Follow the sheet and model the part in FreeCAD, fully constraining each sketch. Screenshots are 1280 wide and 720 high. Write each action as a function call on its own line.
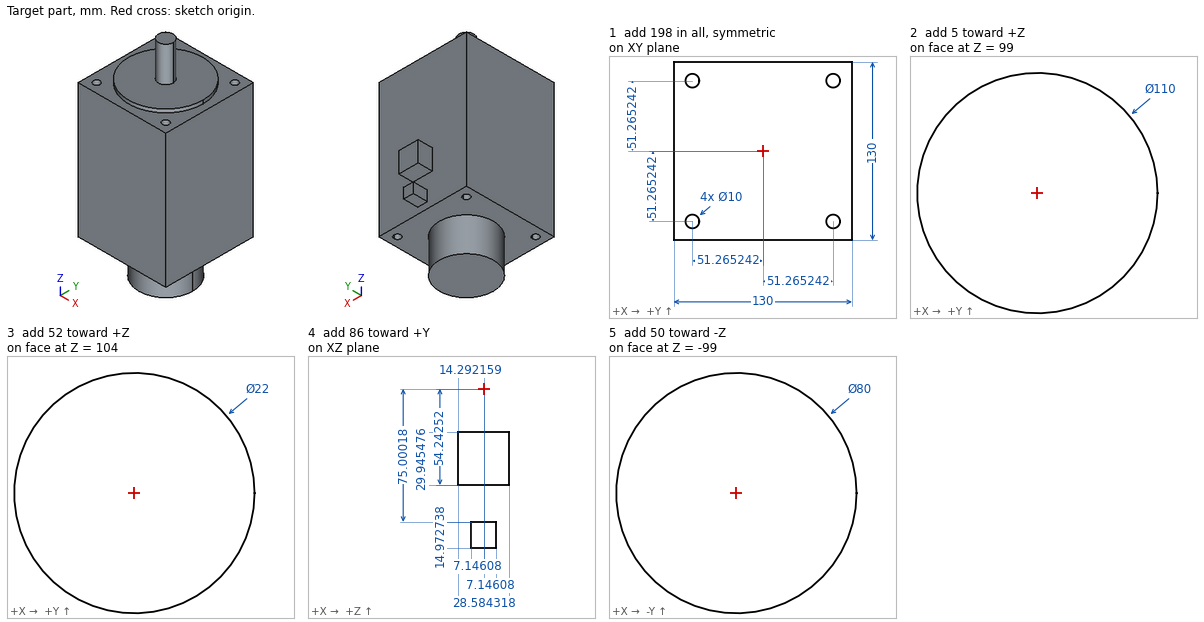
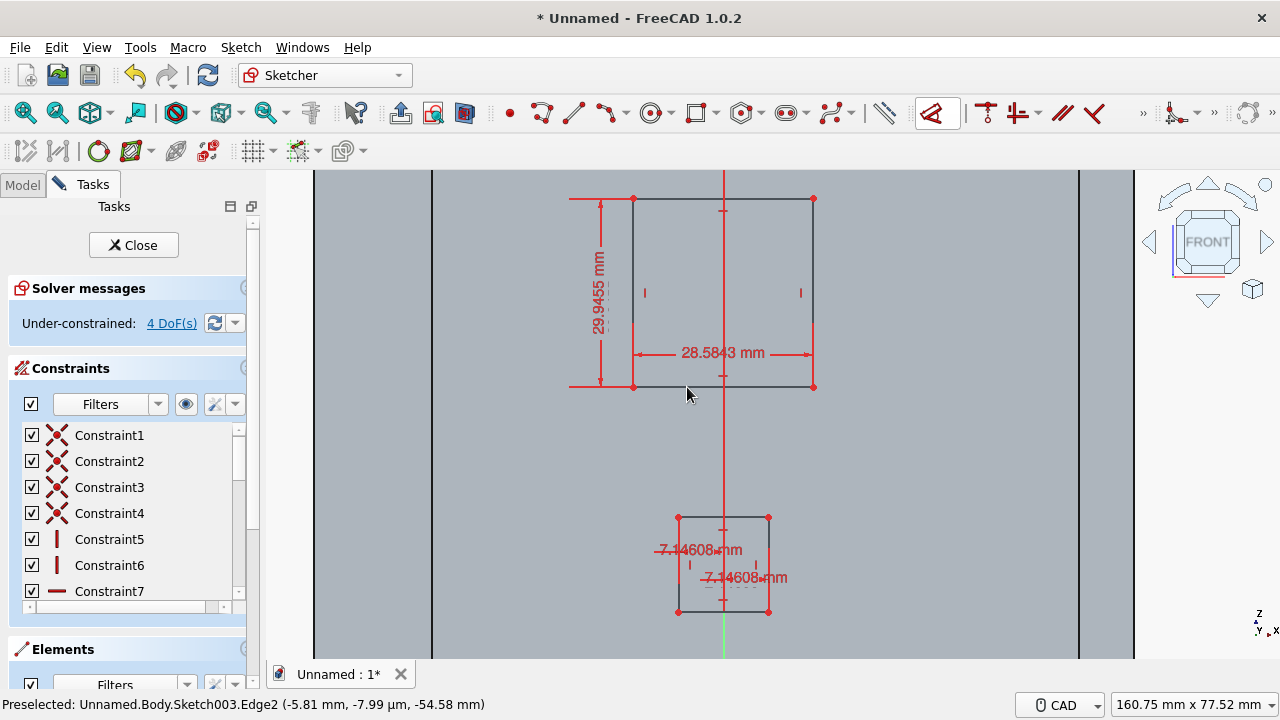
click(679, 584)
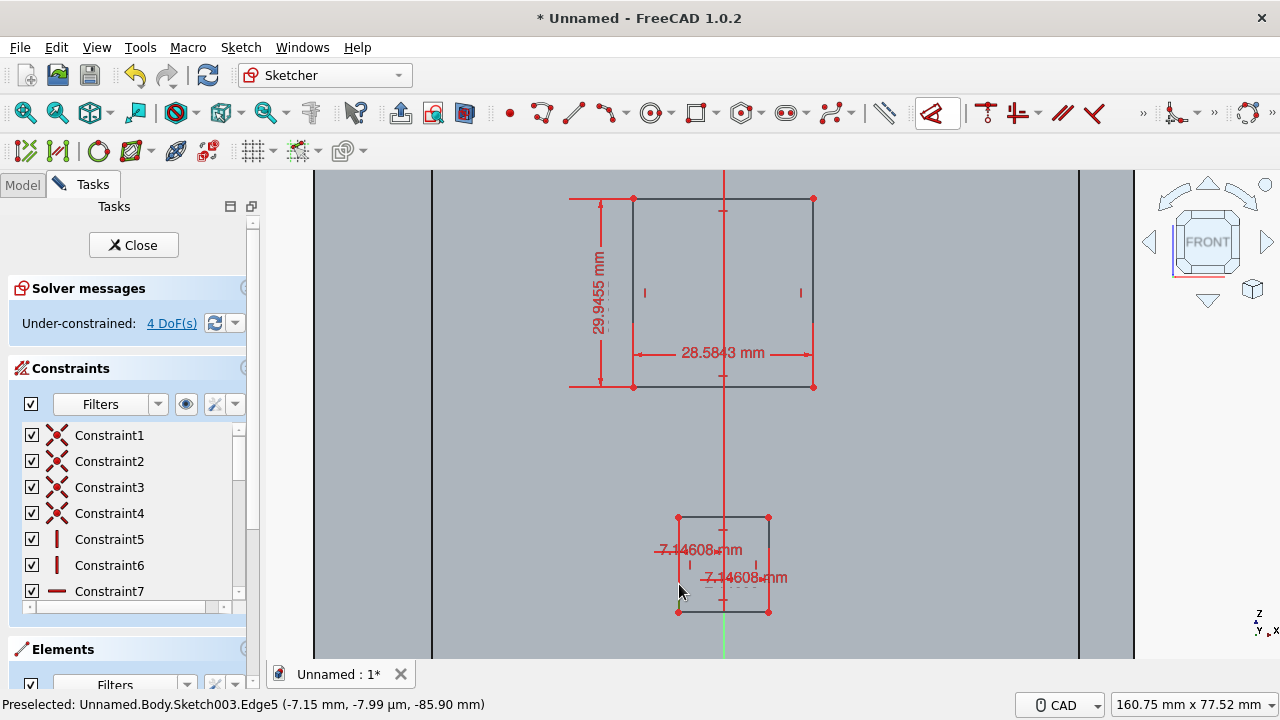
key(i)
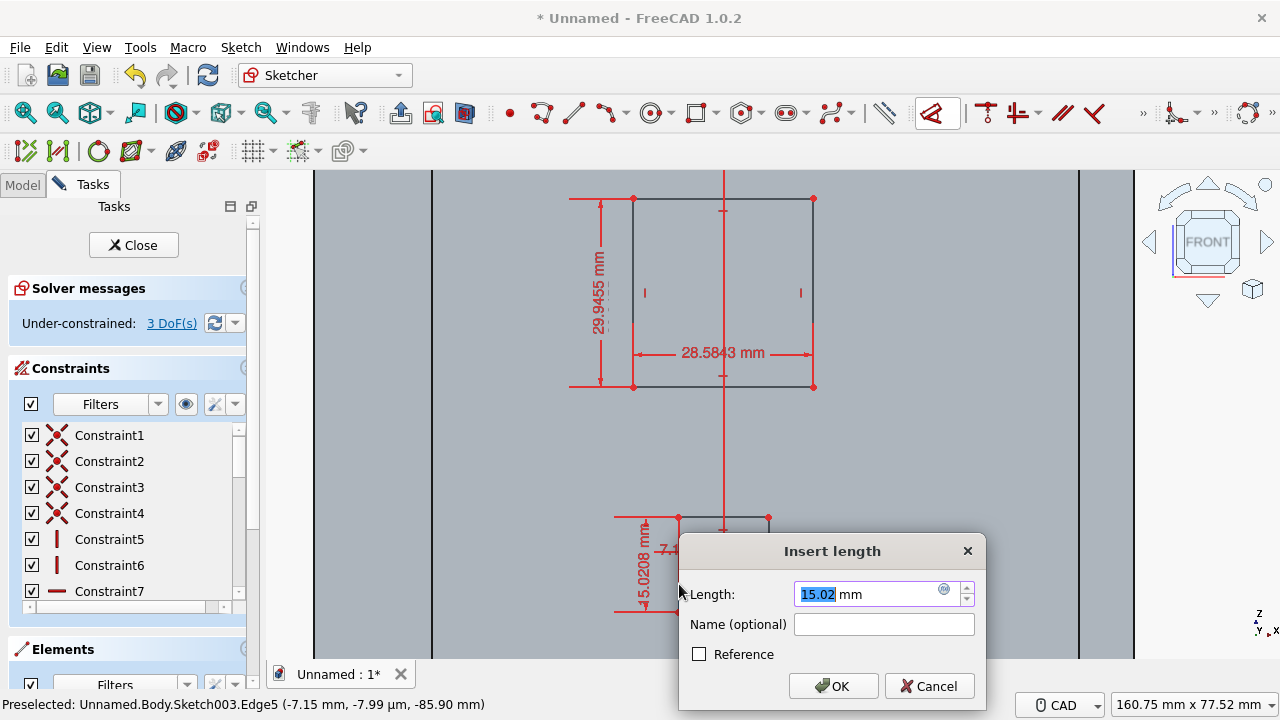
text(14.972738)
key(Return)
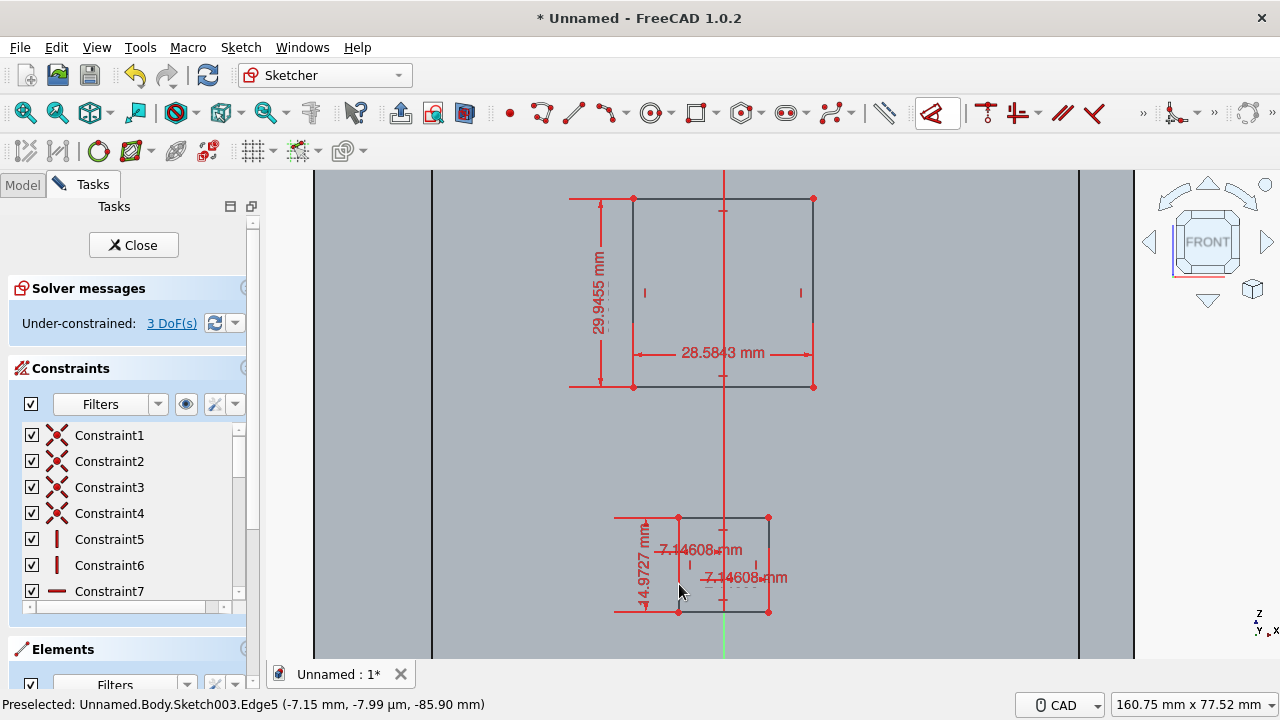
click(633, 387)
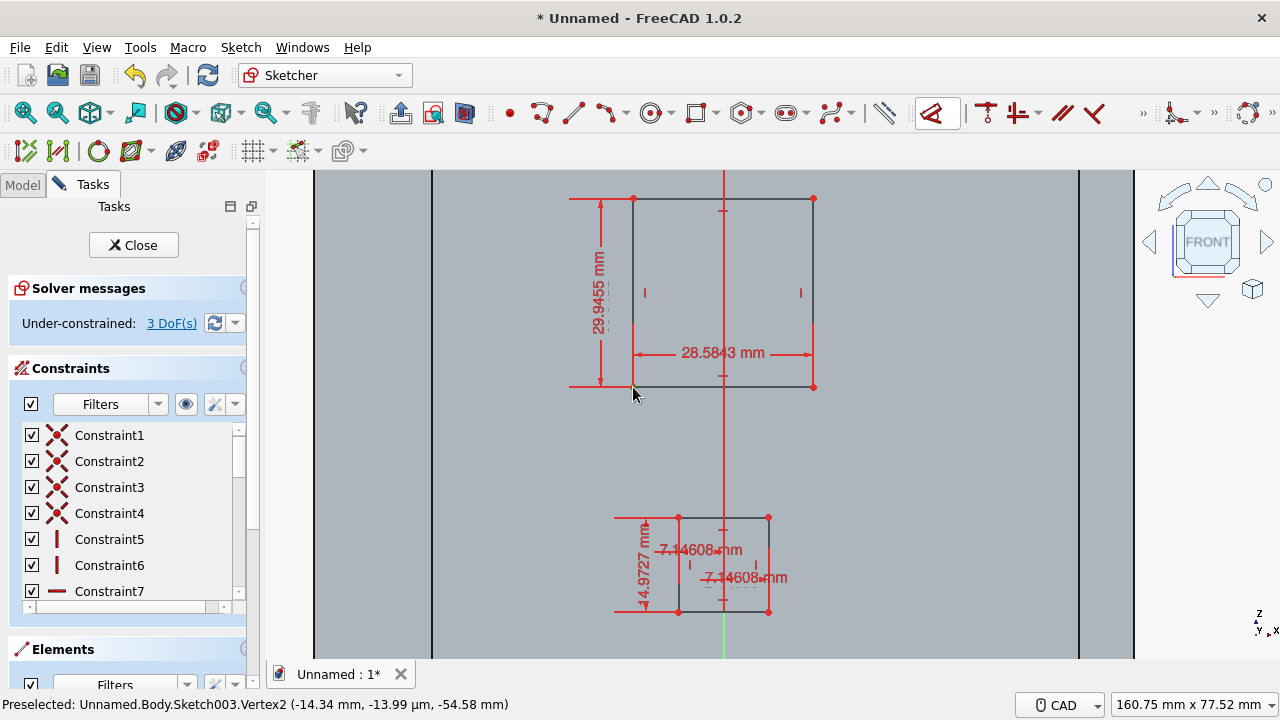
key(i)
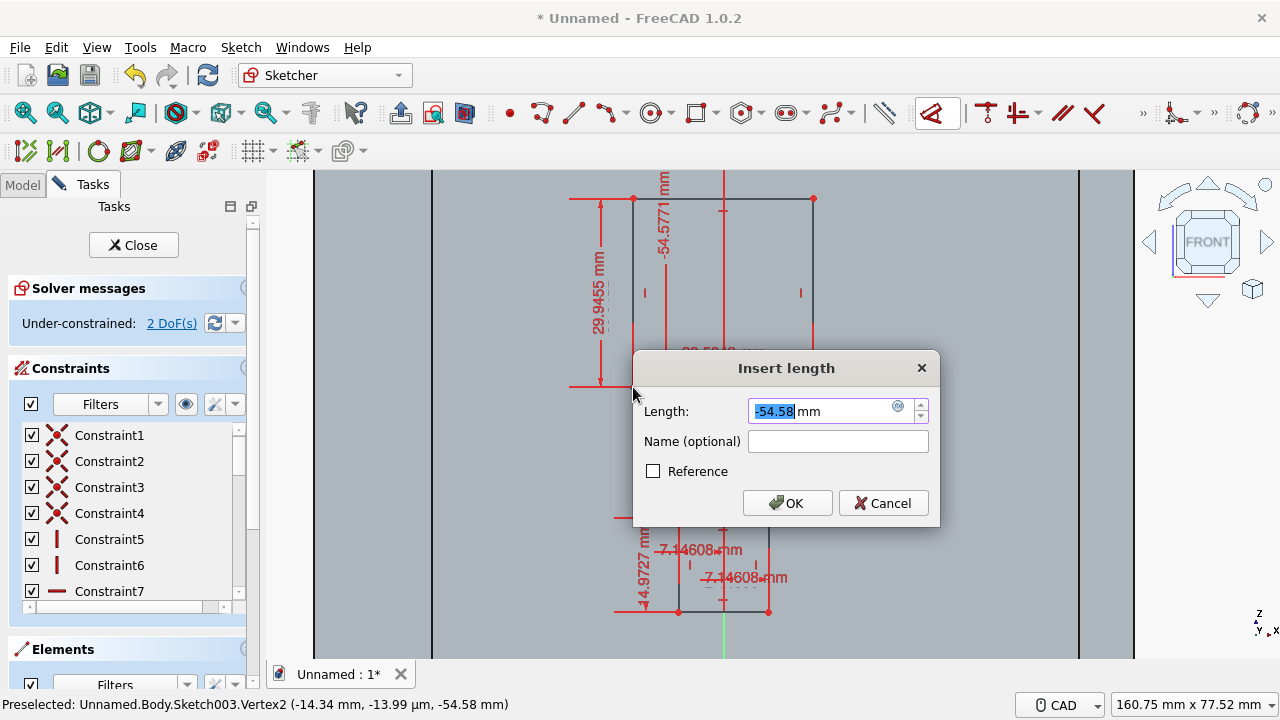
text(-54.24252)
key(Return)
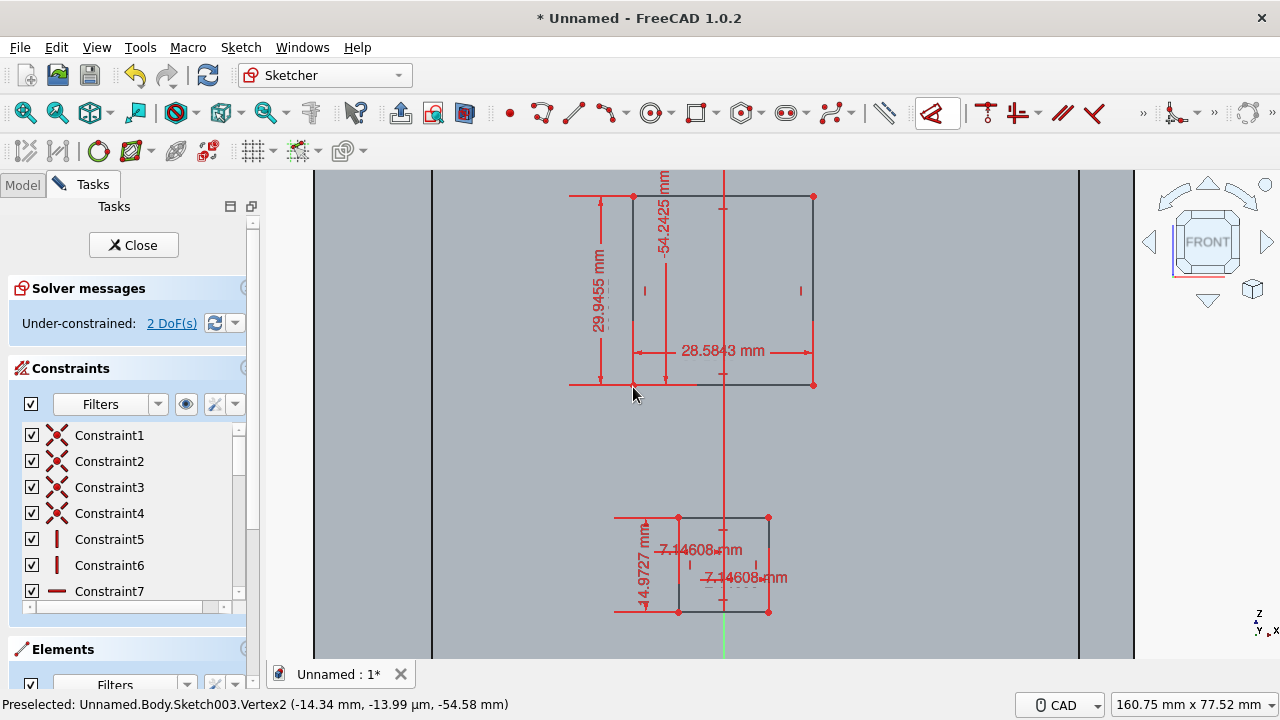
click(679, 518)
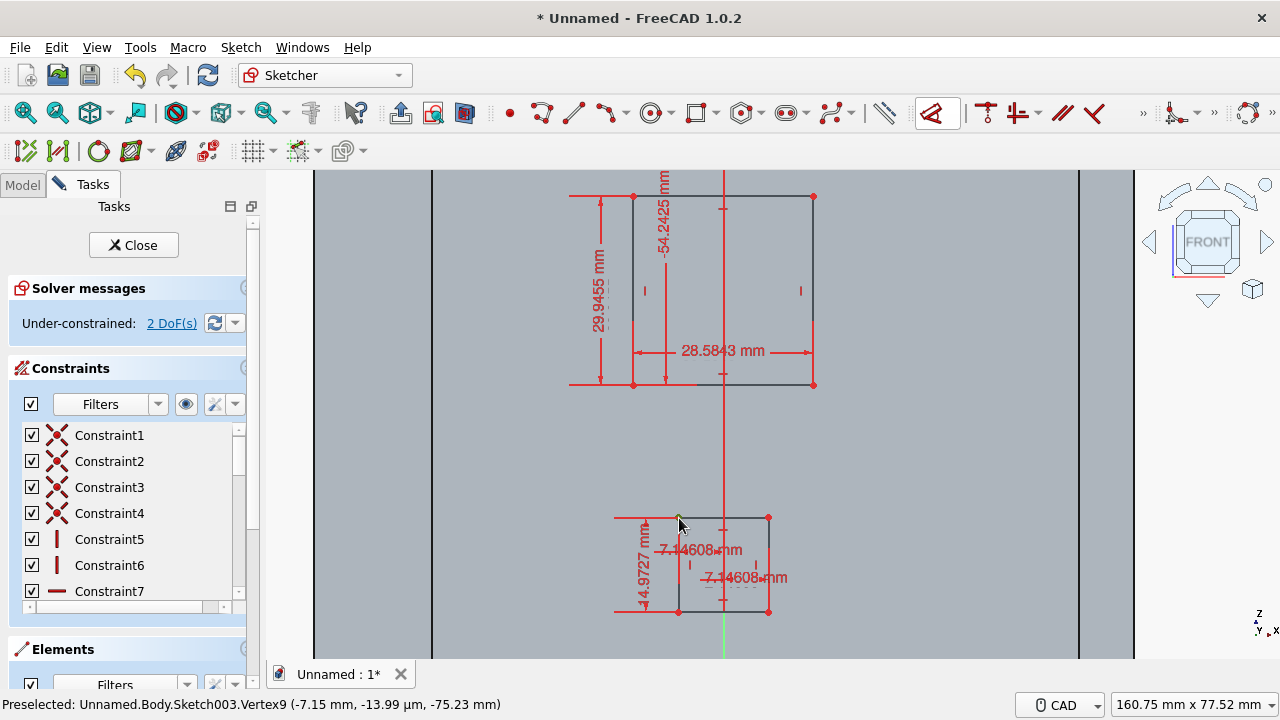
key(i)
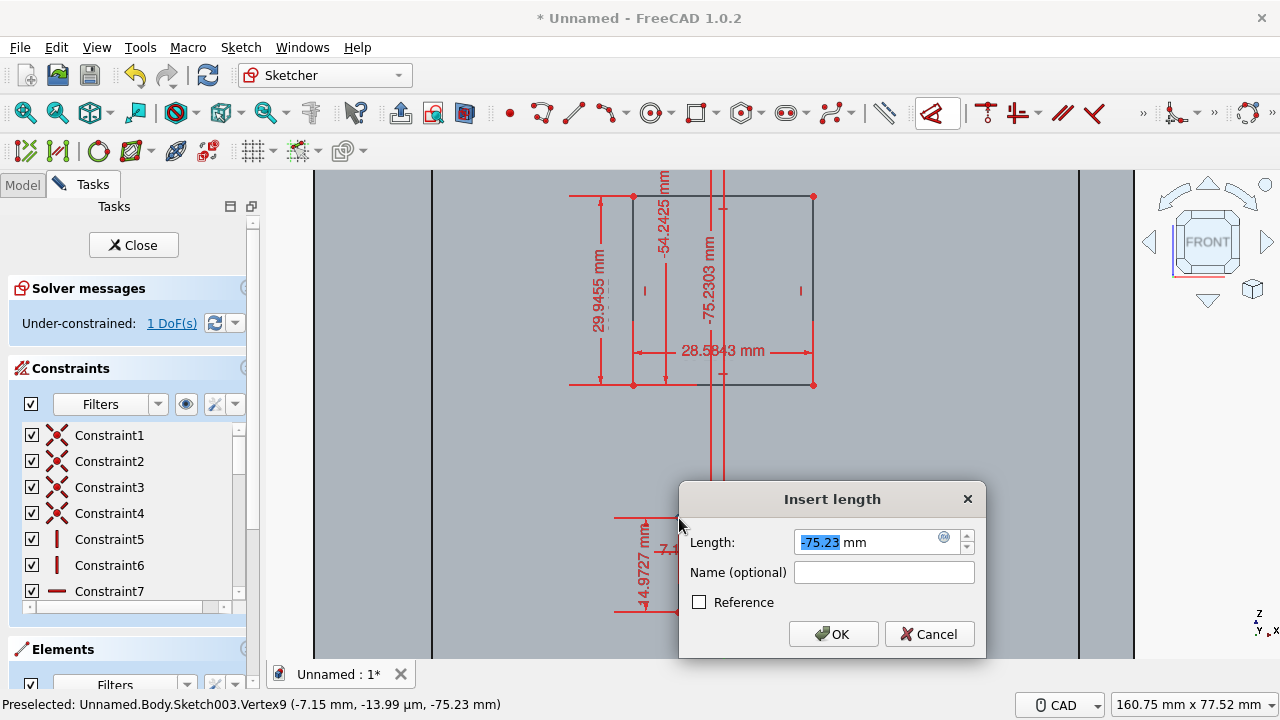
text(-75.00018)
key(Return)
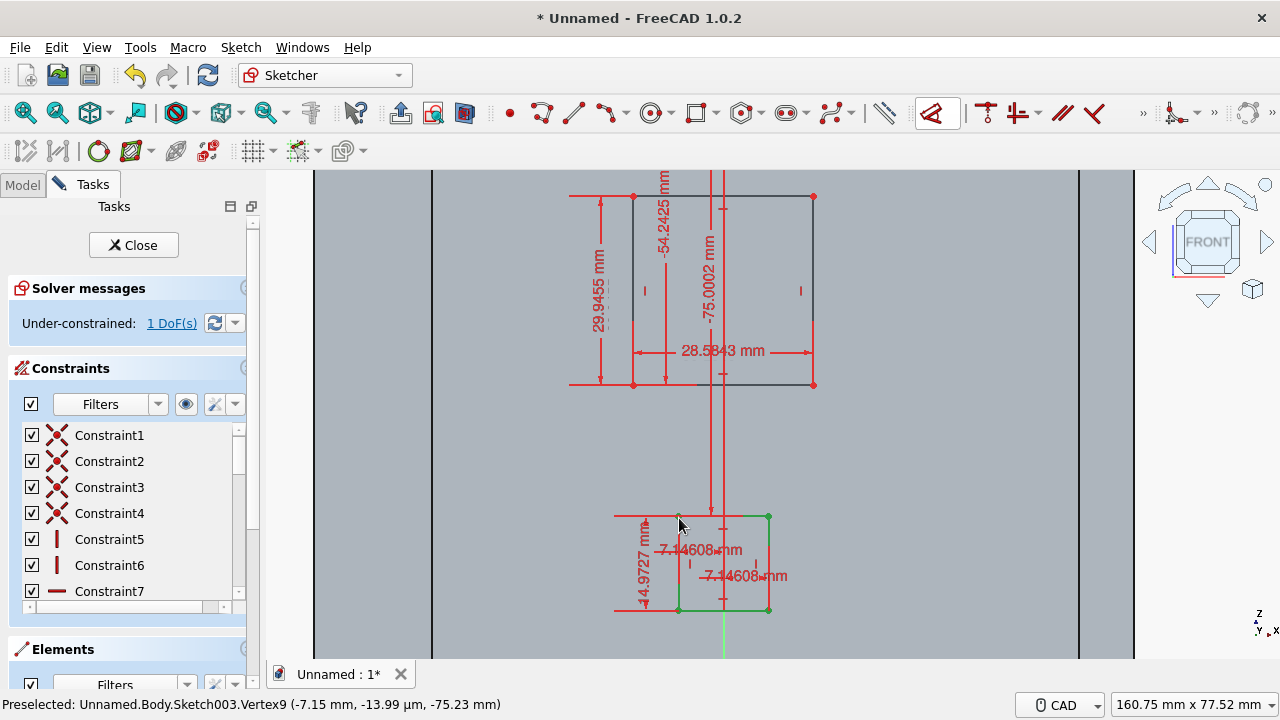
scroll(681, 521, down, 3)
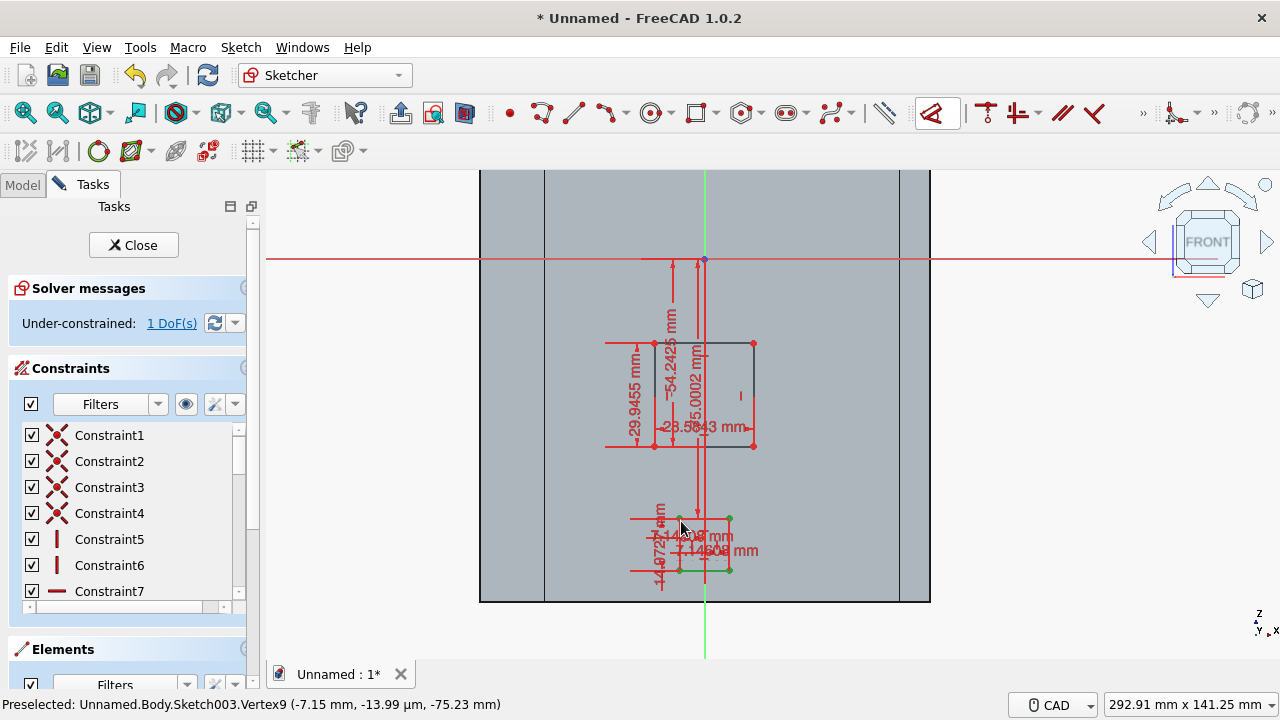
click(655, 343)